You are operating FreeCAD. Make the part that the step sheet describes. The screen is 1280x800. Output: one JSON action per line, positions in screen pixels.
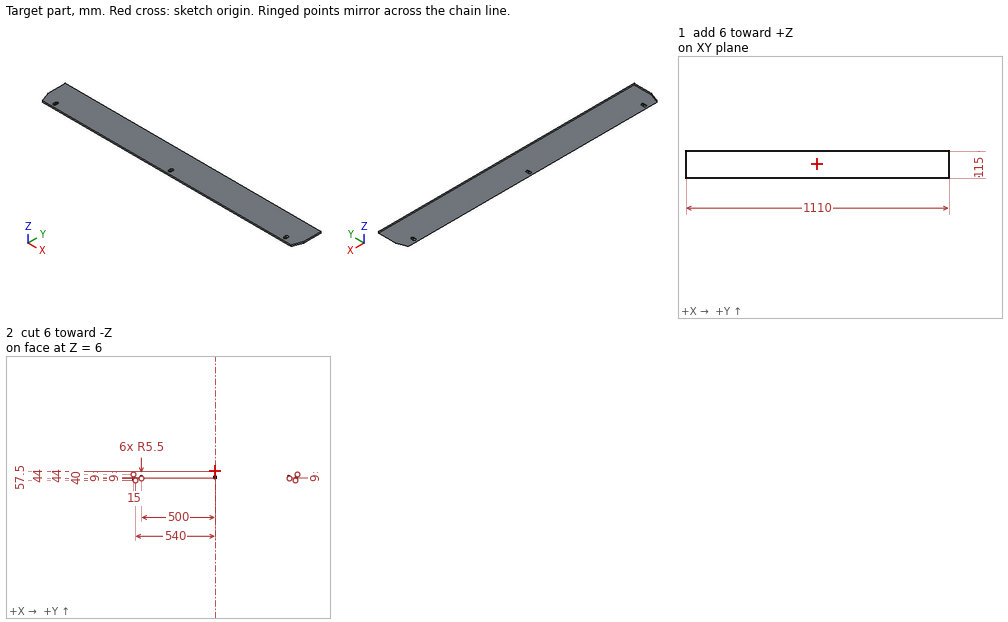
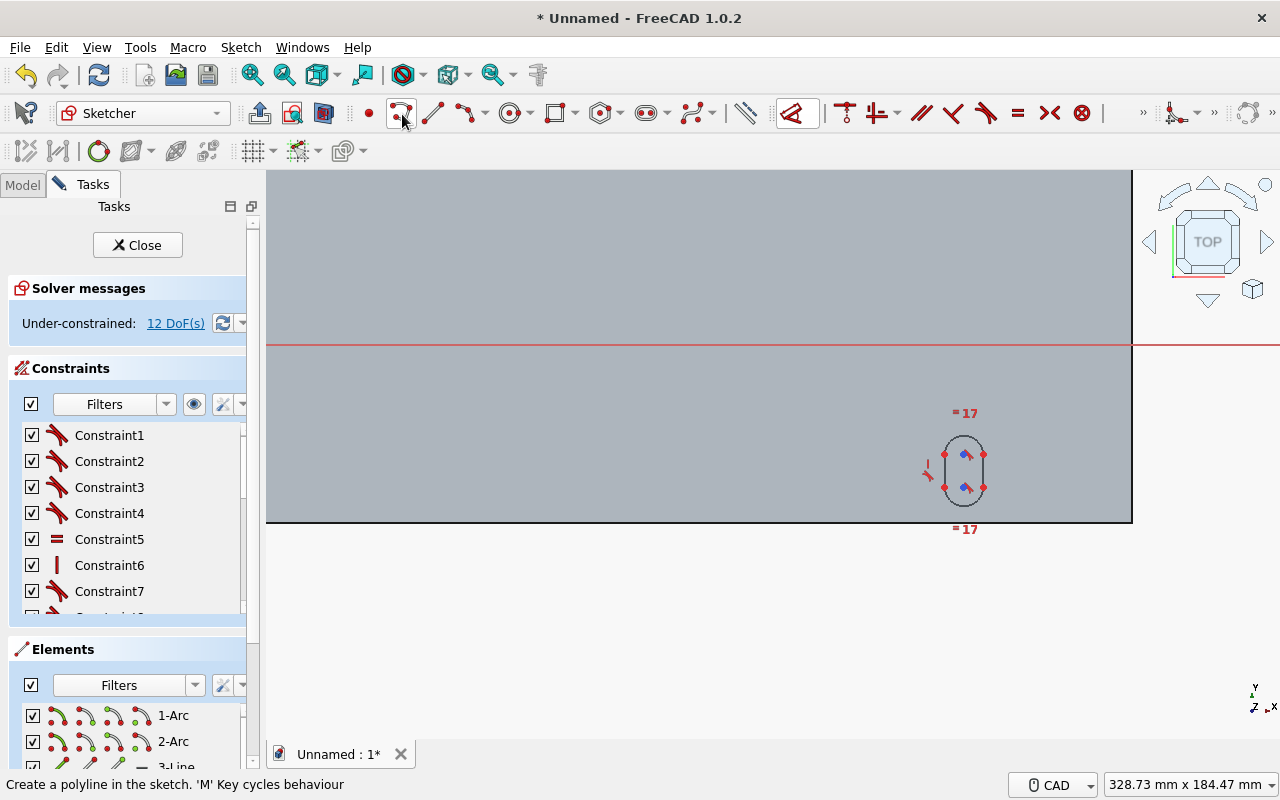
{"action": "scroll", "coordinate": [959, 459], "scroll_direction": "down", "scroll_amount": 9}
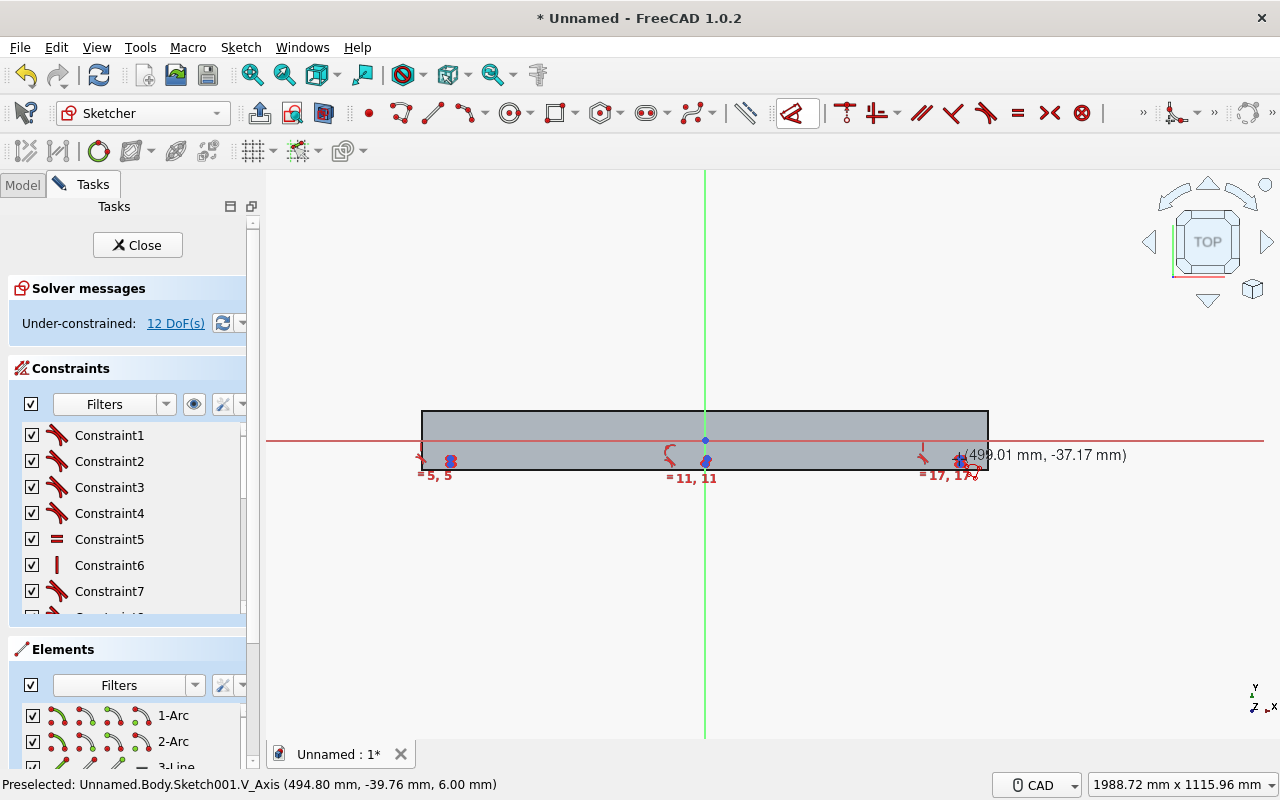
{"action": "left_click", "coordinate": [430, 470]}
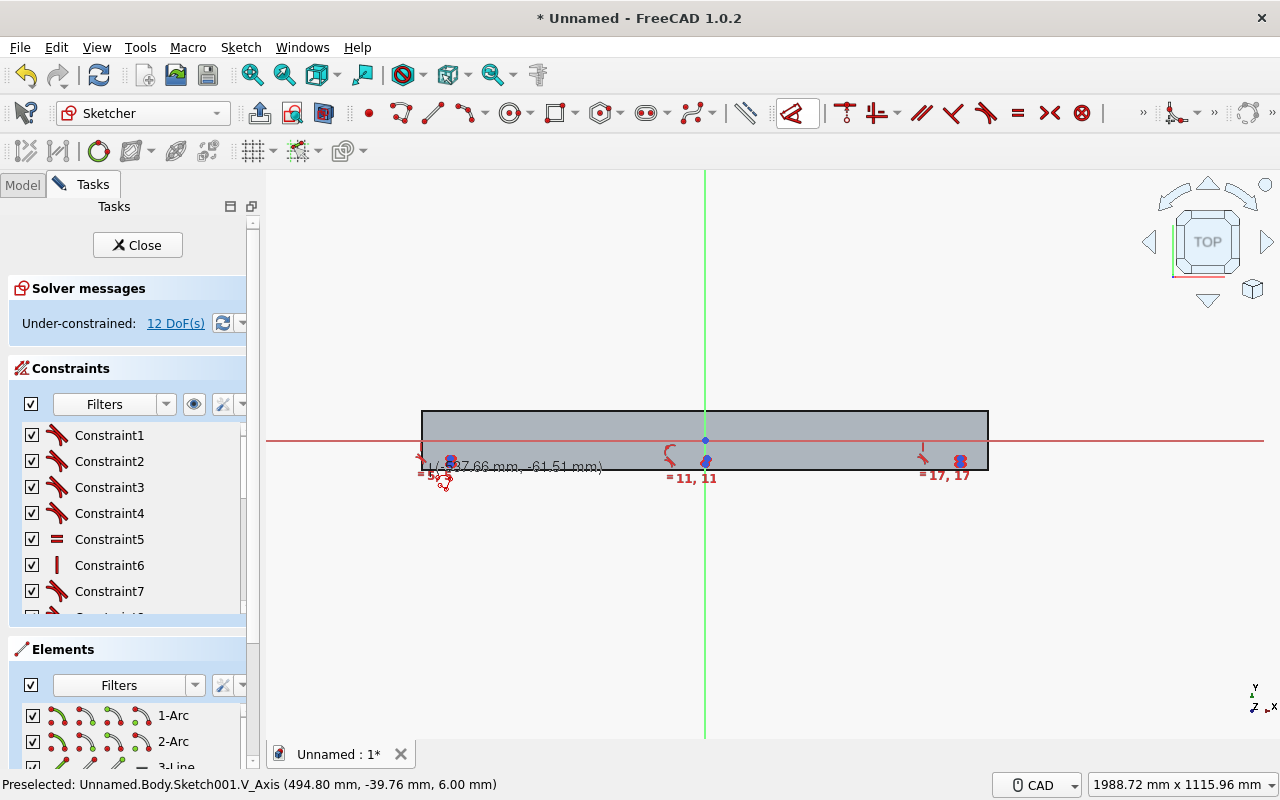
{"action": "scroll", "coordinate": [422, 450], "scroll_direction": "up", "scroll_amount": 3}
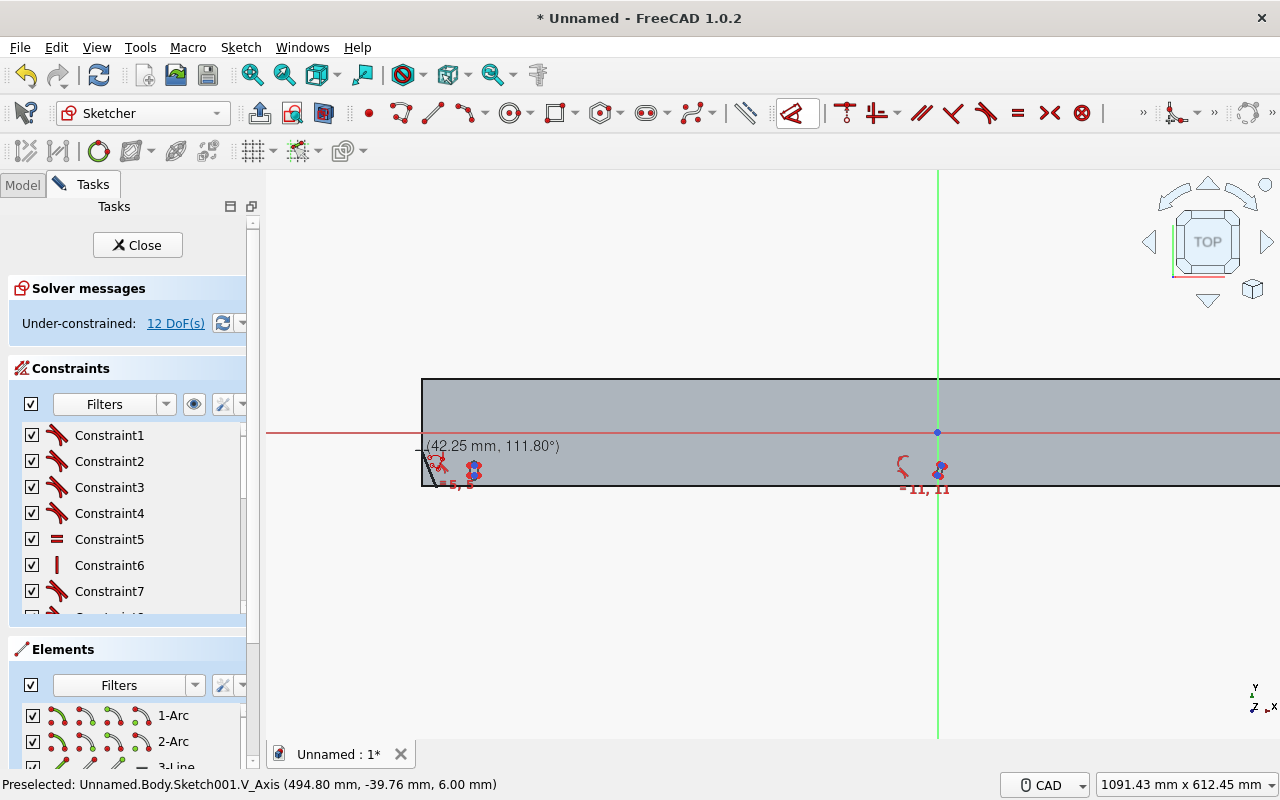
{"action": "left_click", "coordinate": [422, 449]}
{"action": "left_click", "coordinate": [422, 486]}
{"action": "left_click", "coordinate": [436, 488]}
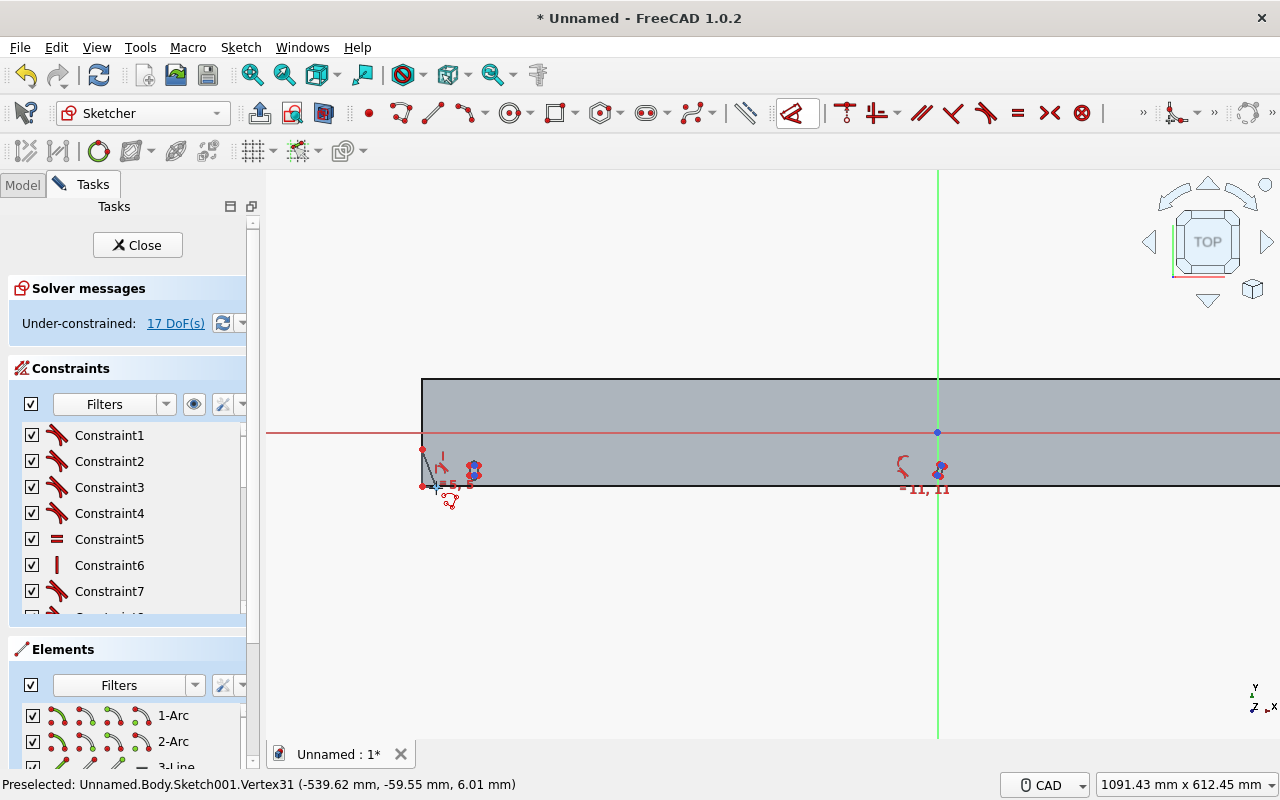
{"action": "scroll", "coordinate": [421, 449], "scroll_direction": "down", "scroll_amount": 3}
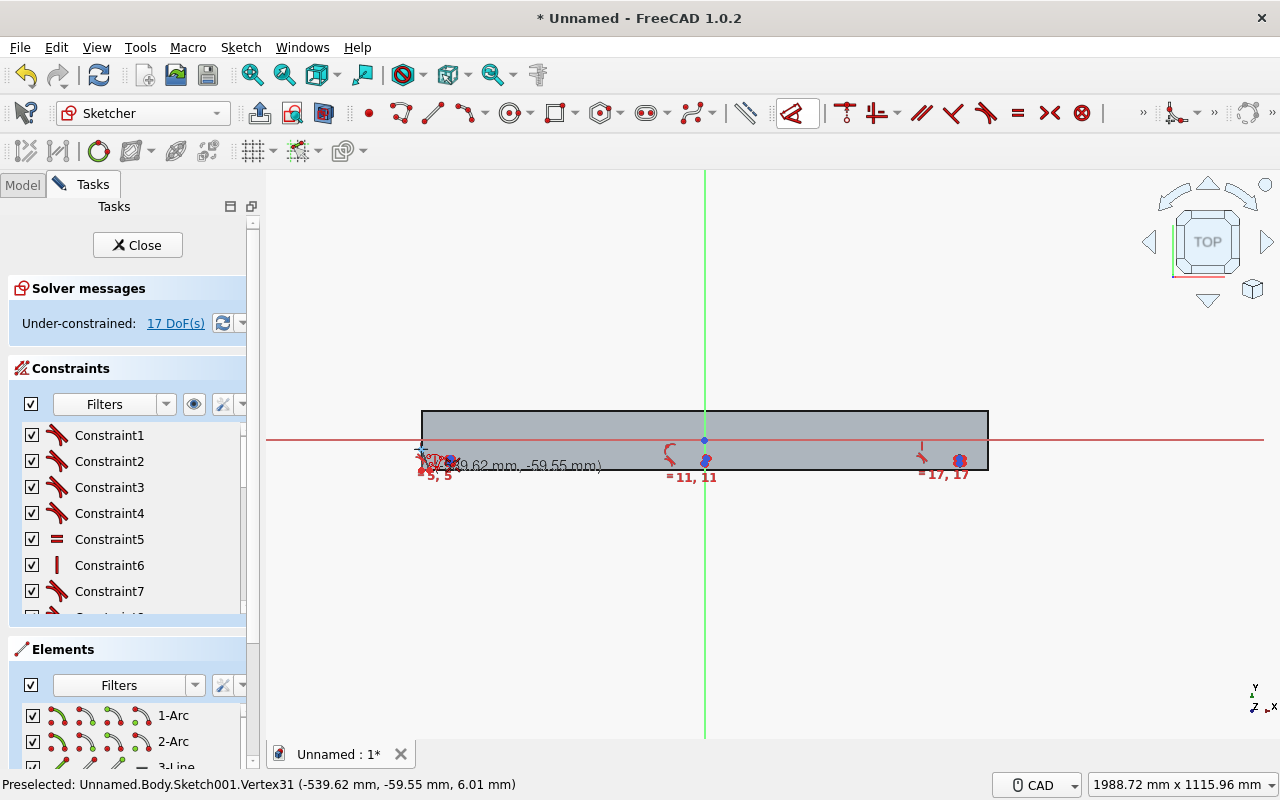
{"action": "left_click", "coordinate": [980, 470]}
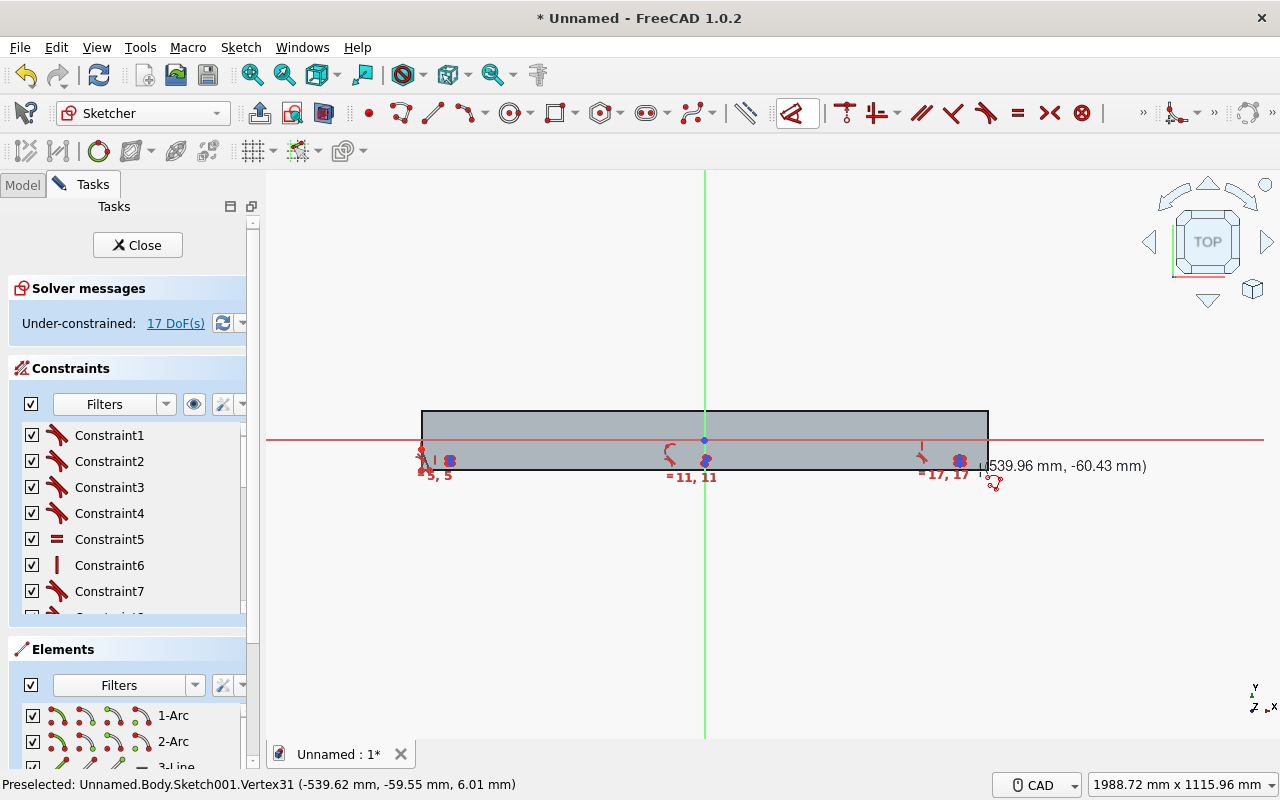
{"action": "scroll", "coordinate": [988, 470], "scroll_direction": "up", "scroll_amount": 4}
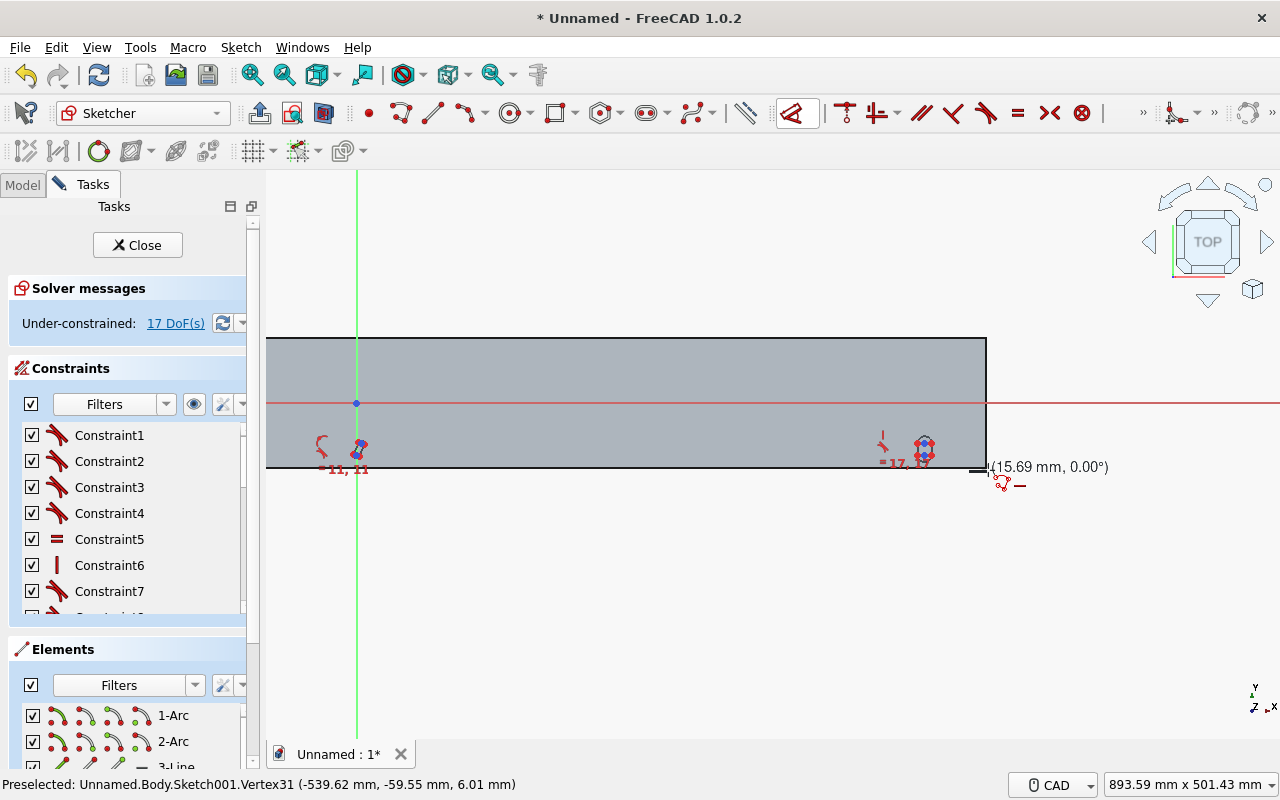
{"action": "left_click", "coordinate": [986, 469]}
{"action": "left_click", "coordinate": [986, 423]}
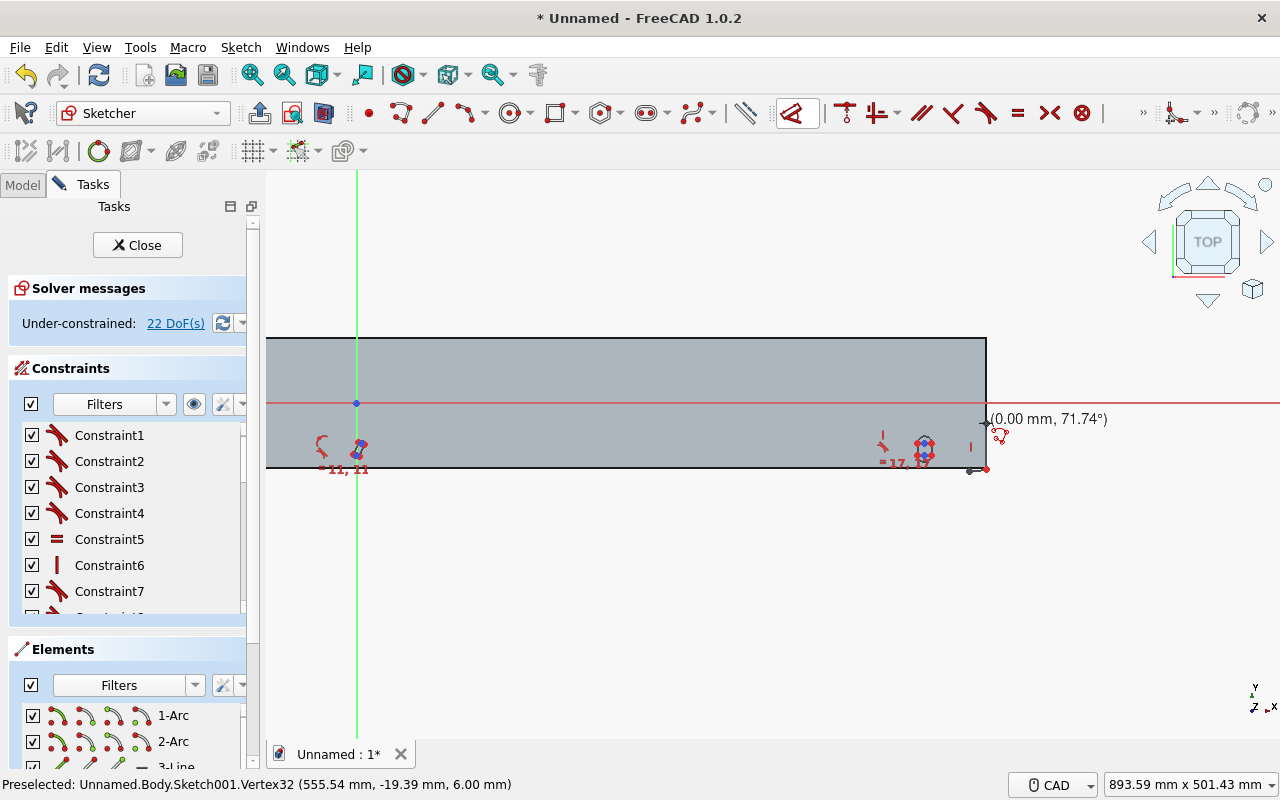
{"action": "scroll", "coordinate": [969, 468], "scroll_direction": "up", "scroll_amount": 4}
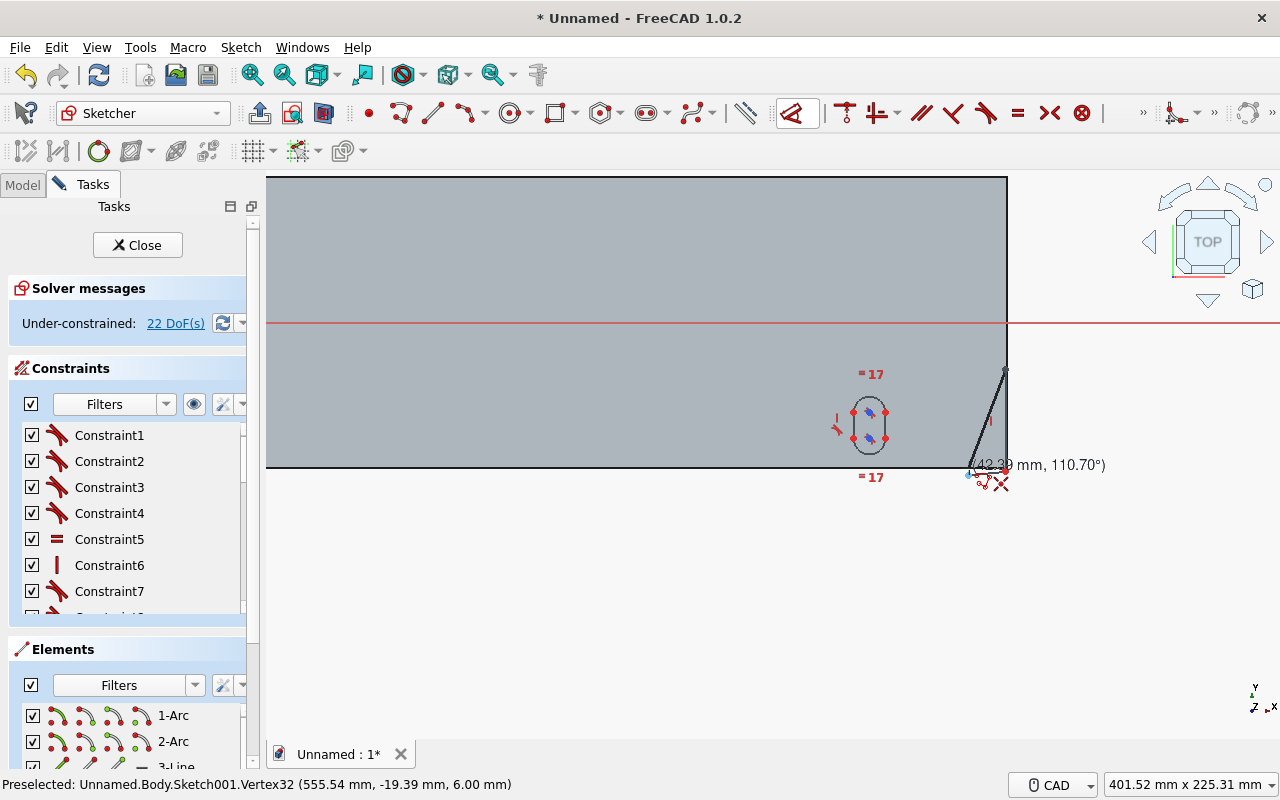
{"action": "left_click", "coordinate": [969, 475]}
{"action": "key", "text": "Escape"}
{"action": "key", "text": "Escape"}